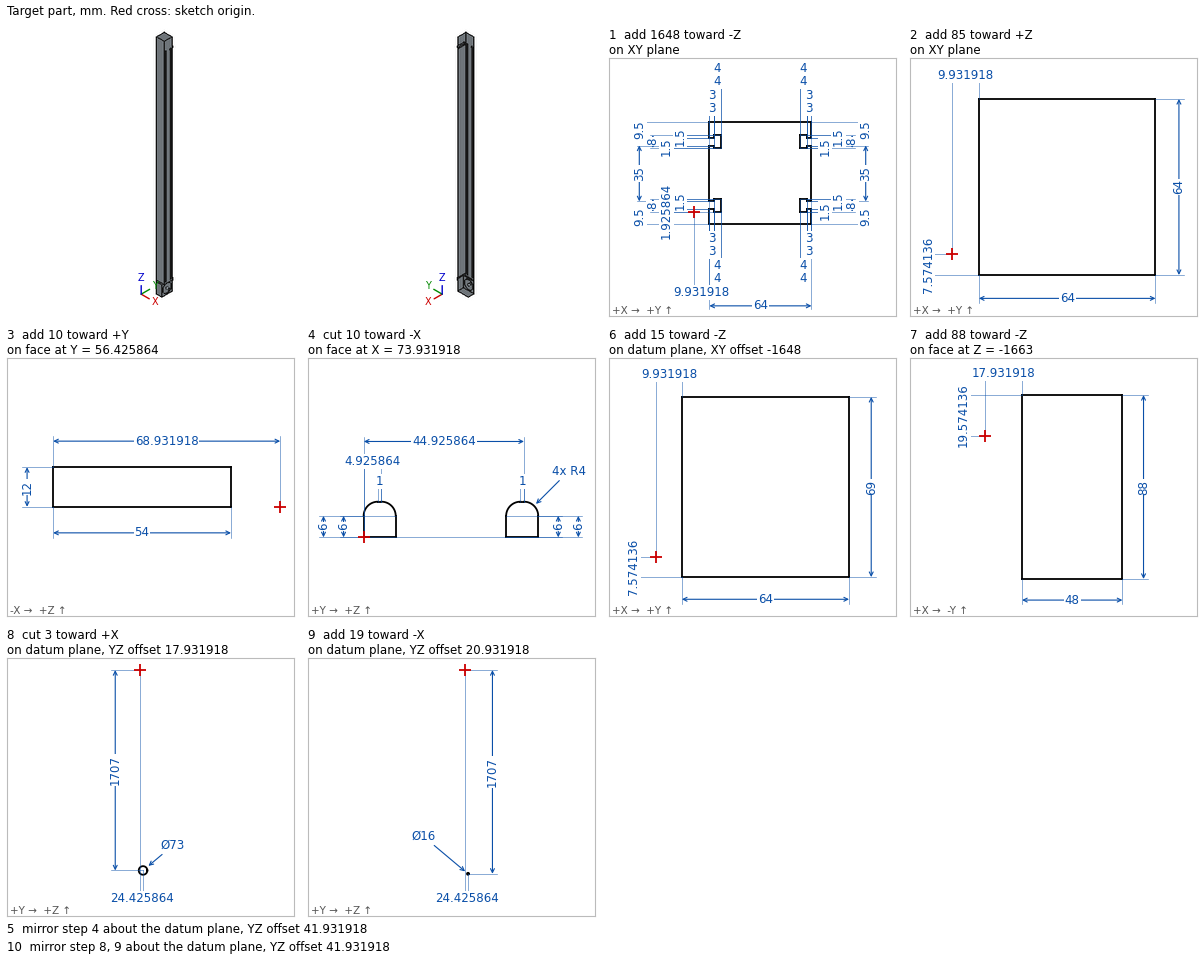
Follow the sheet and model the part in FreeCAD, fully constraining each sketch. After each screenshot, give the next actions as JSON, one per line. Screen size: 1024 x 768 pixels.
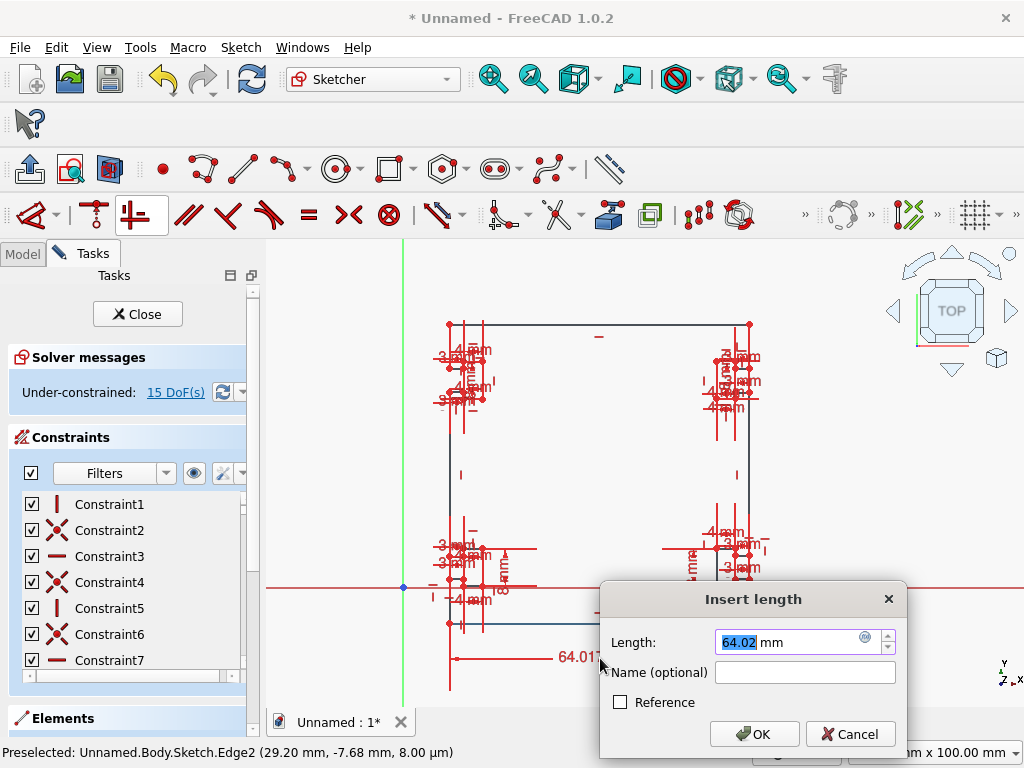
{"action": "type", "text": "64"}
{"action": "key", "text": "Return"}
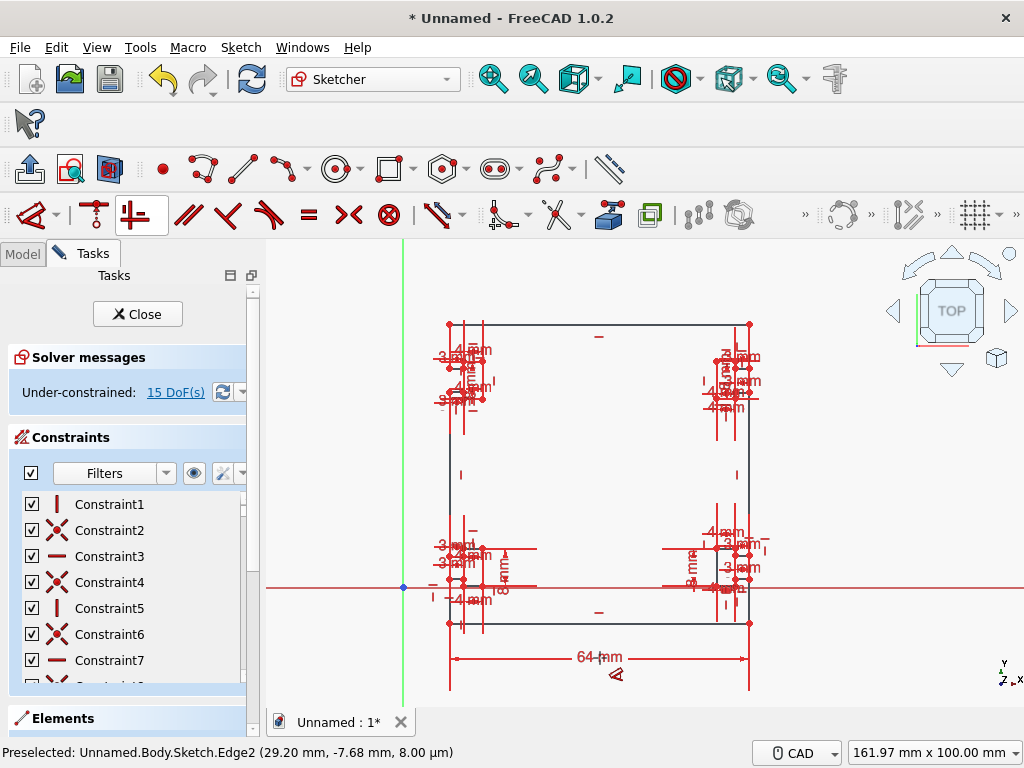
{"action": "left_click", "coordinate": [749, 507]}
{"action": "left_click", "coordinate": [783, 474]}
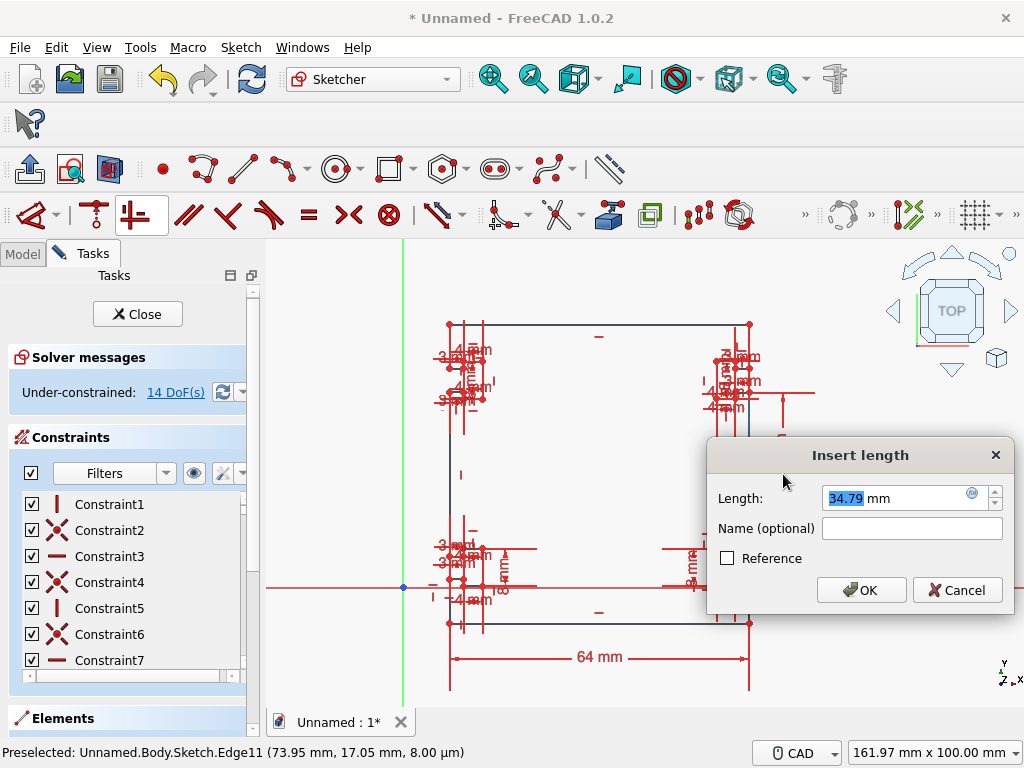
{"action": "type", "text": "35"}
{"action": "key", "text": "Return"}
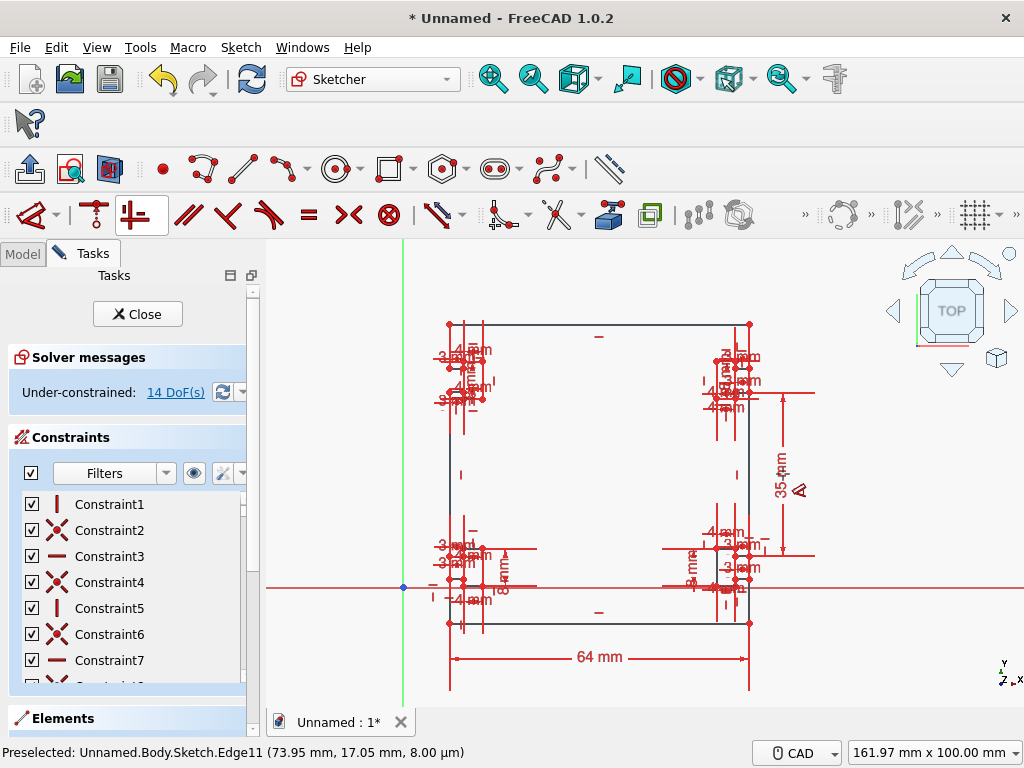
{"action": "left_click", "coordinate": [450, 441]}
{"action": "left_click", "coordinate": [484, 474]}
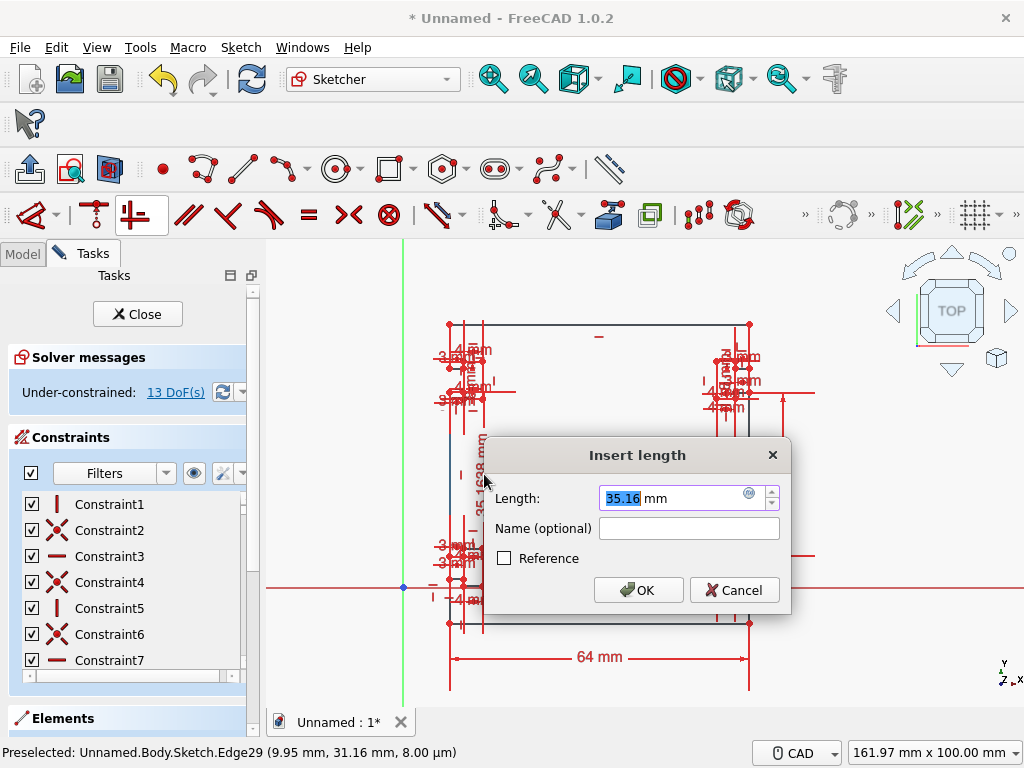
{"action": "type", "text": "35"}
{"action": "key", "text": "Return"}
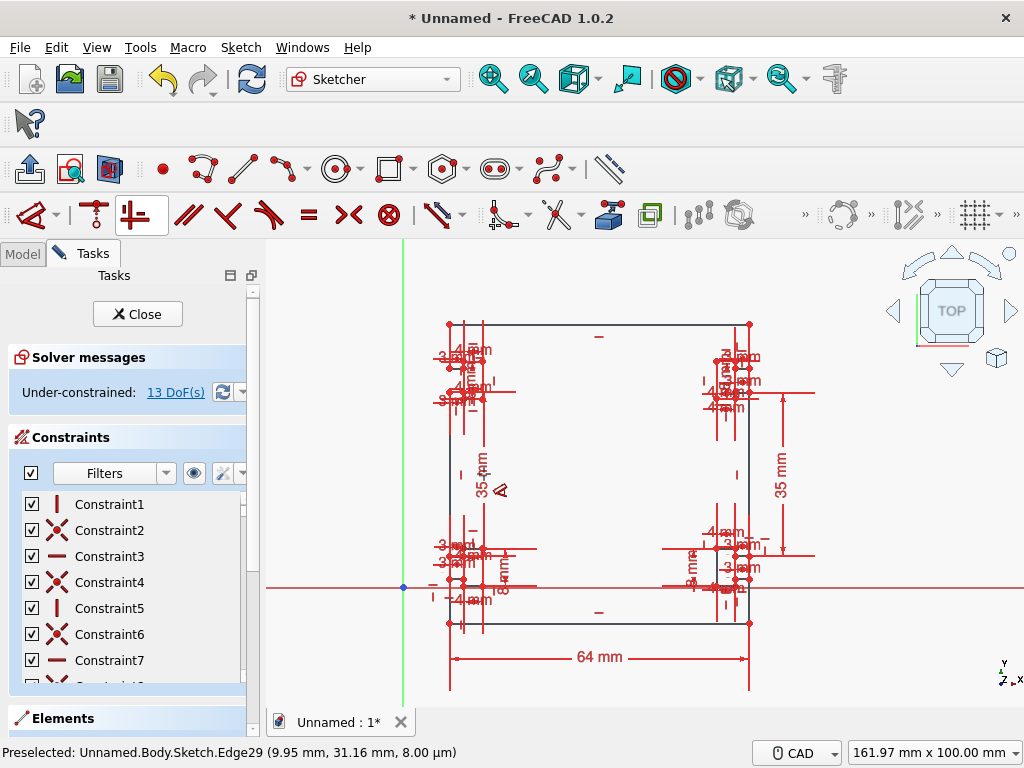
{"action": "left_click", "coordinate": [450, 610]}
{"action": "left_click", "coordinate": [368, 601]}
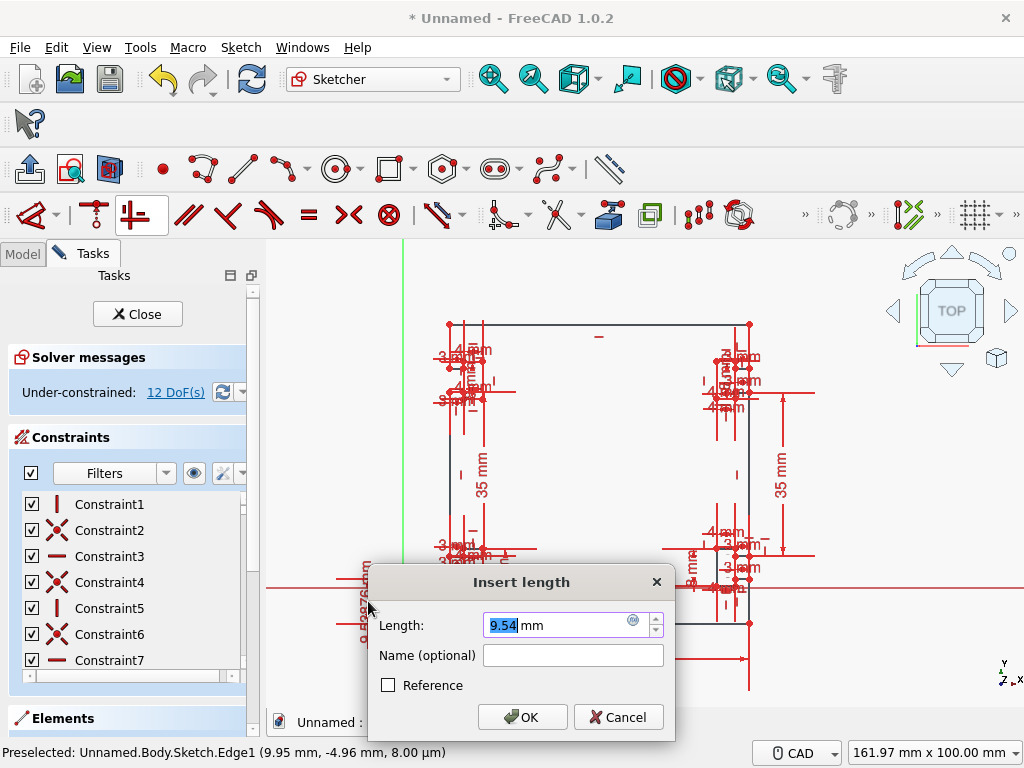
{"action": "type", "text": "9.5"}
{"action": "key", "text": "Return"}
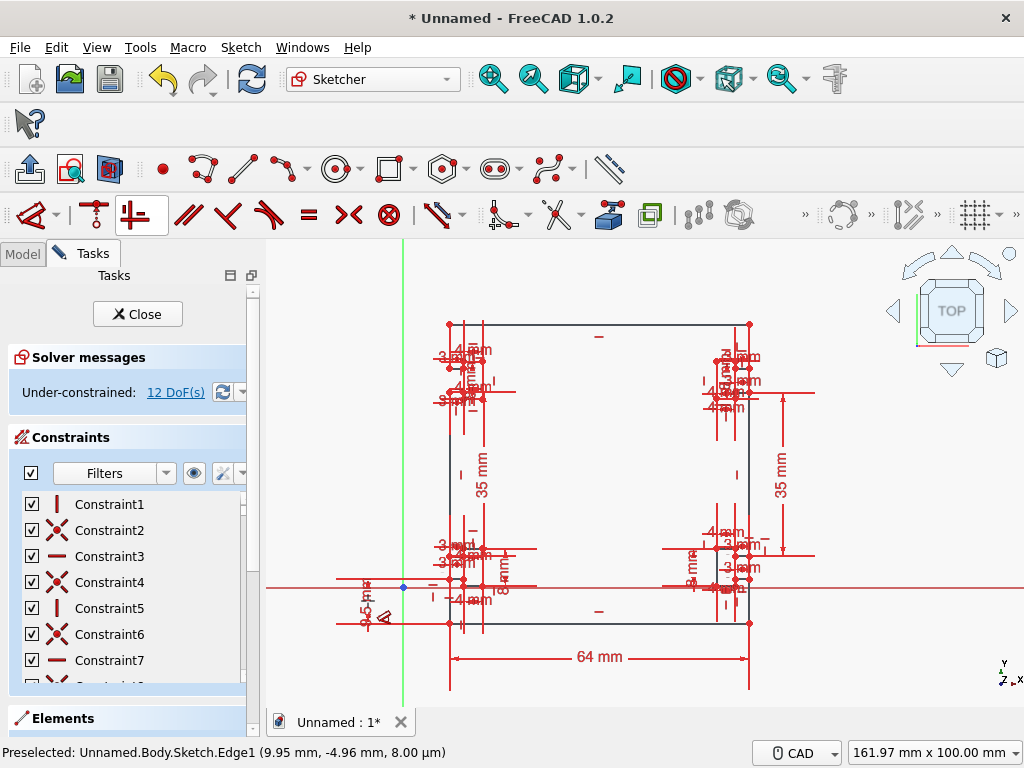
{"action": "left_click", "coordinate": [749, 610]}
{"action": "left_click", "coordinate": [783, 612]}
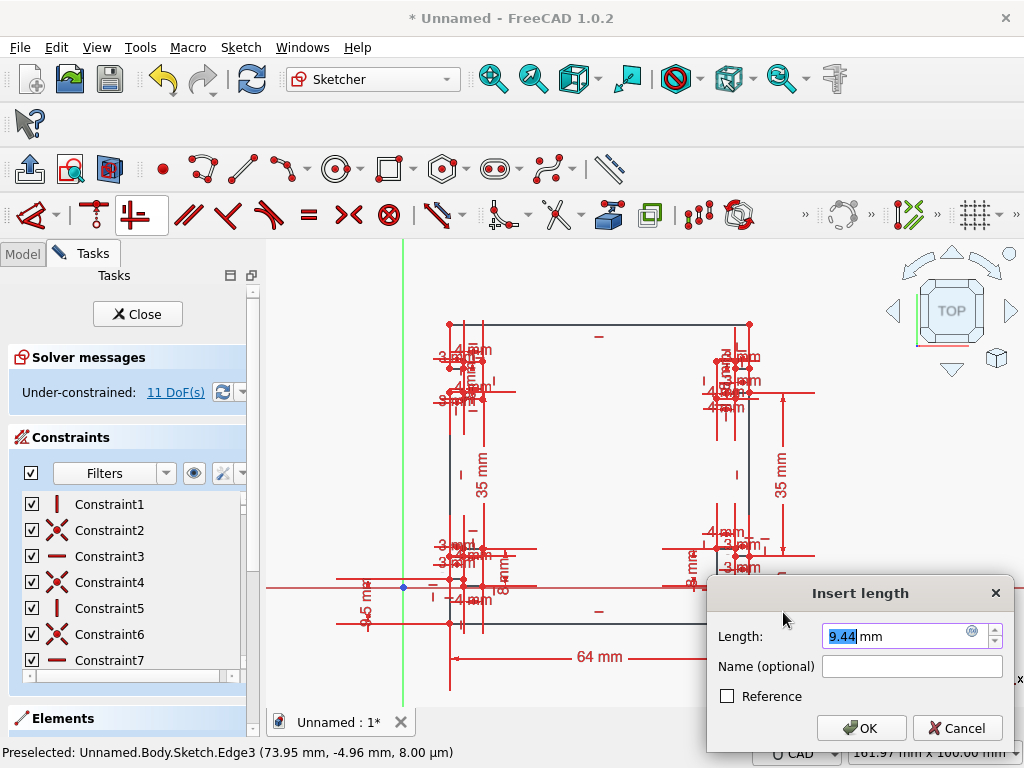
{"action": "type", "text": "9.5"}
{"action": "key", "text": "Return"}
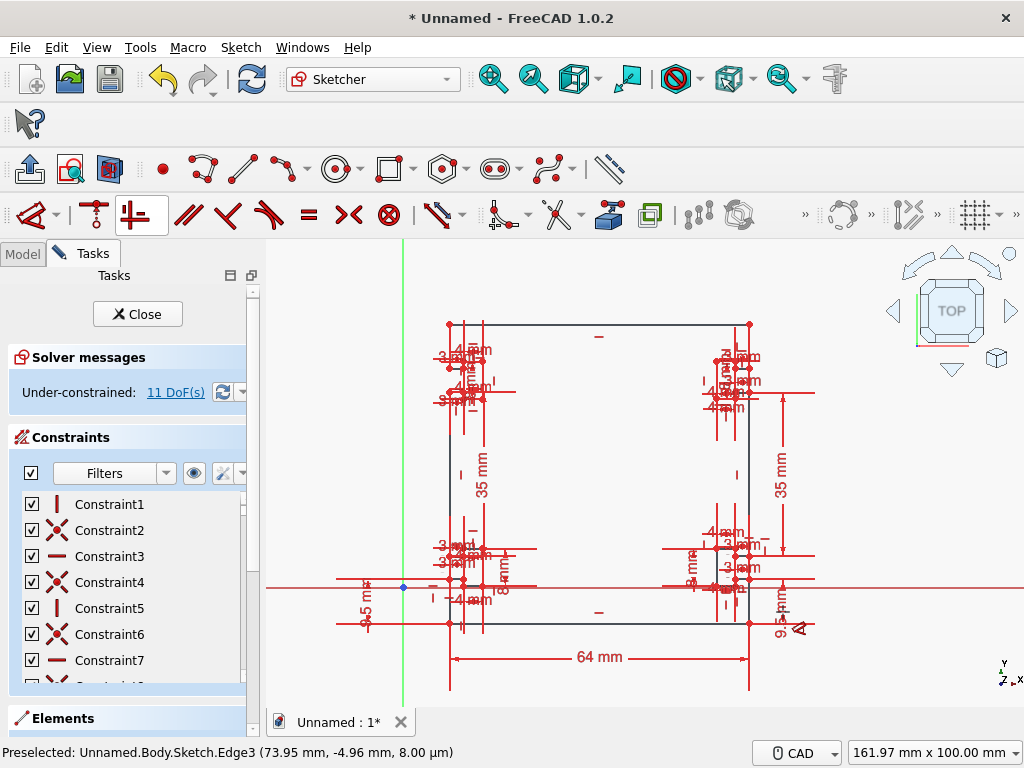
{"action": "scroll", "coordinate": [735, 583], "scroll_direction": "up", "scroll_amount": 9}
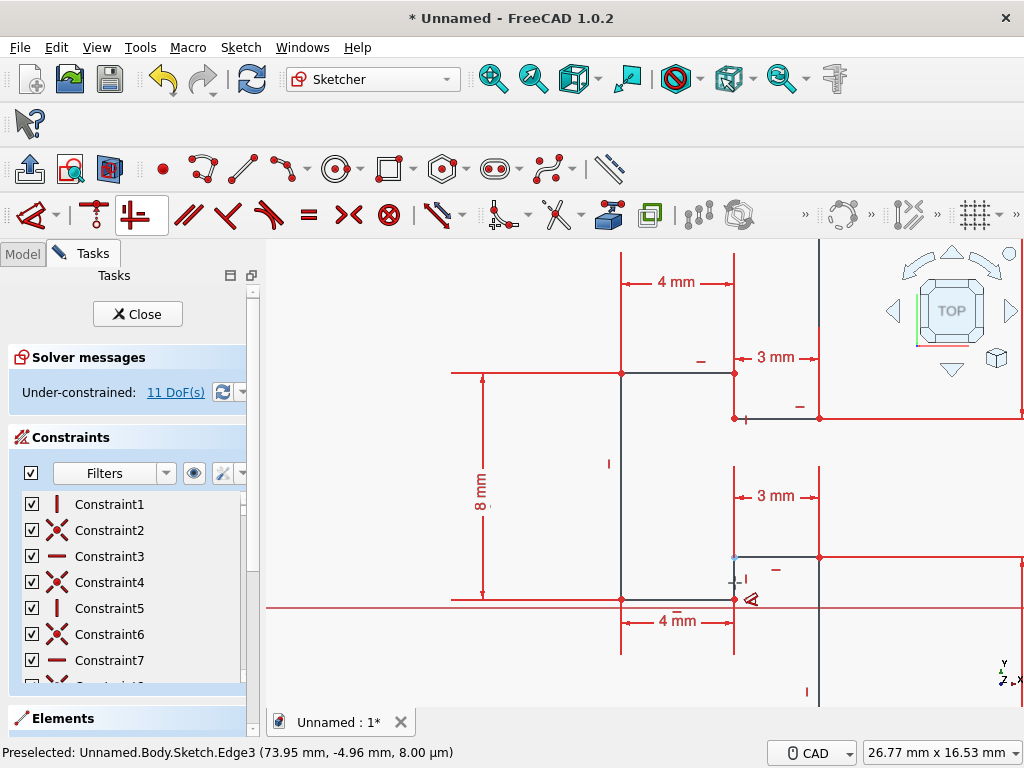
{"action": "left_click", "coordinate": [734, 579]}
{"action": "left_click", "coordinate": [768, 579]}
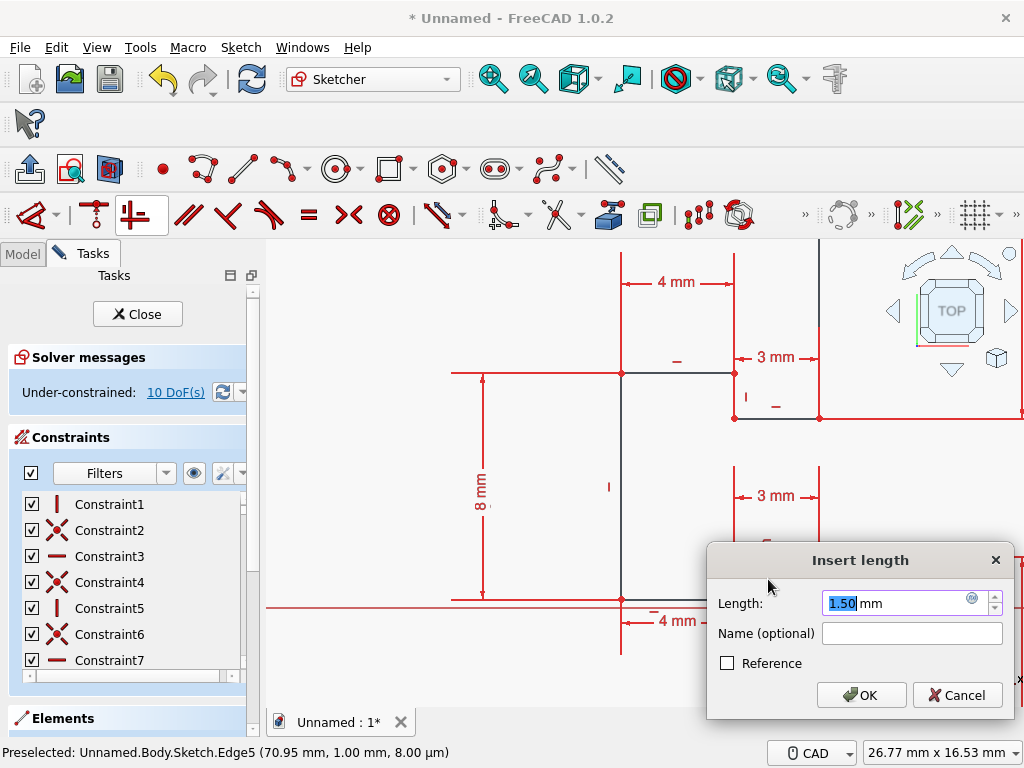
{"action": "type", "text": "1.5"}
{"action": "key", "text": "Return"}